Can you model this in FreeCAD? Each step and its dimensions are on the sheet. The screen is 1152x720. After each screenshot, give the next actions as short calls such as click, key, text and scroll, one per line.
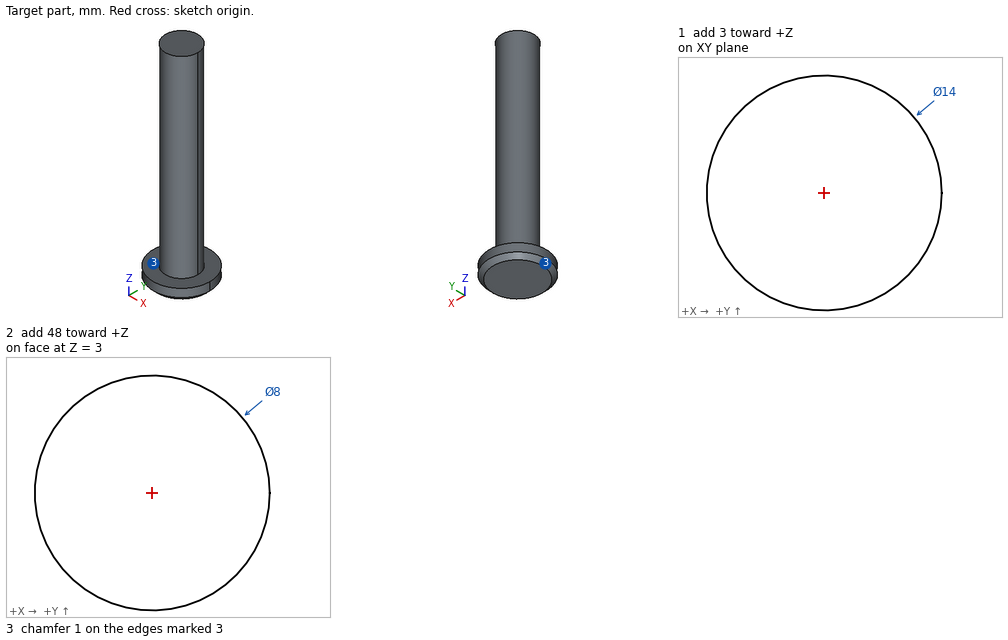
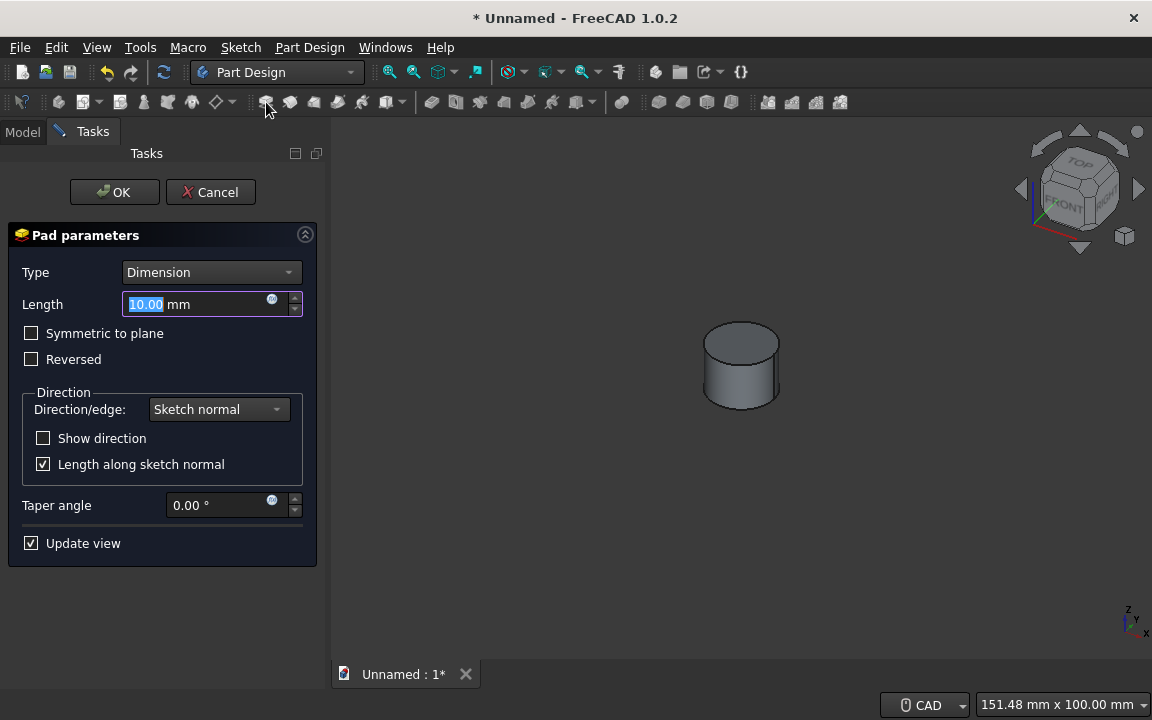
text(3)
key(Tab)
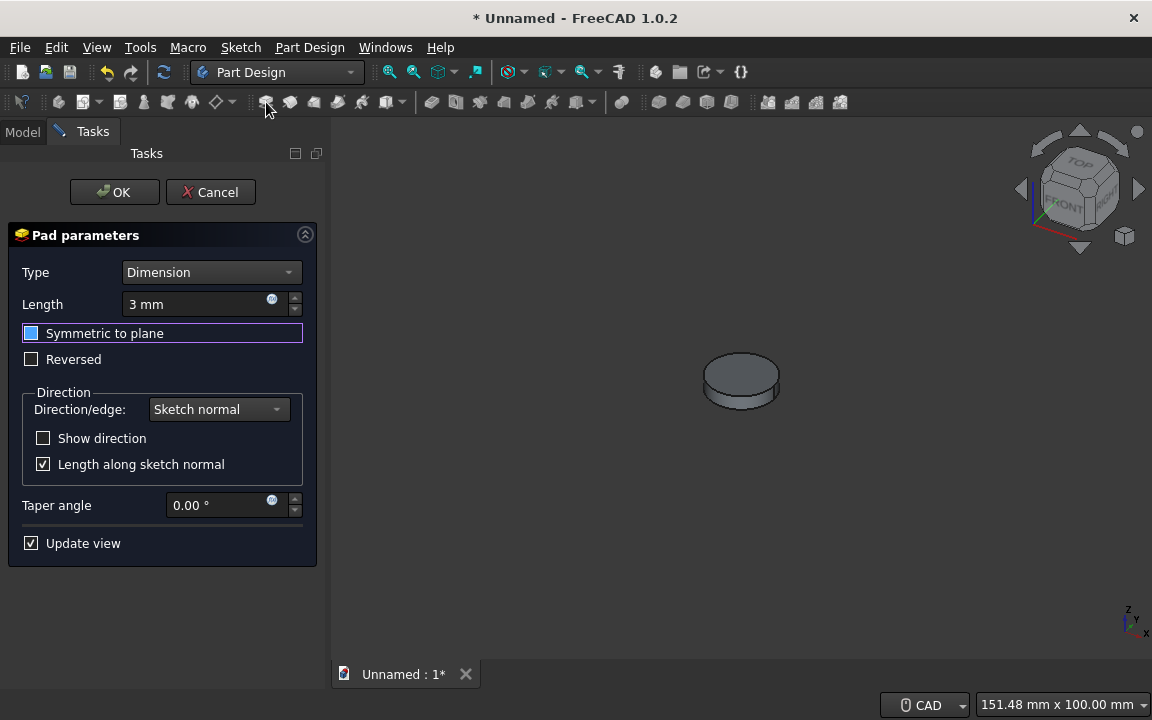
click(115, 192)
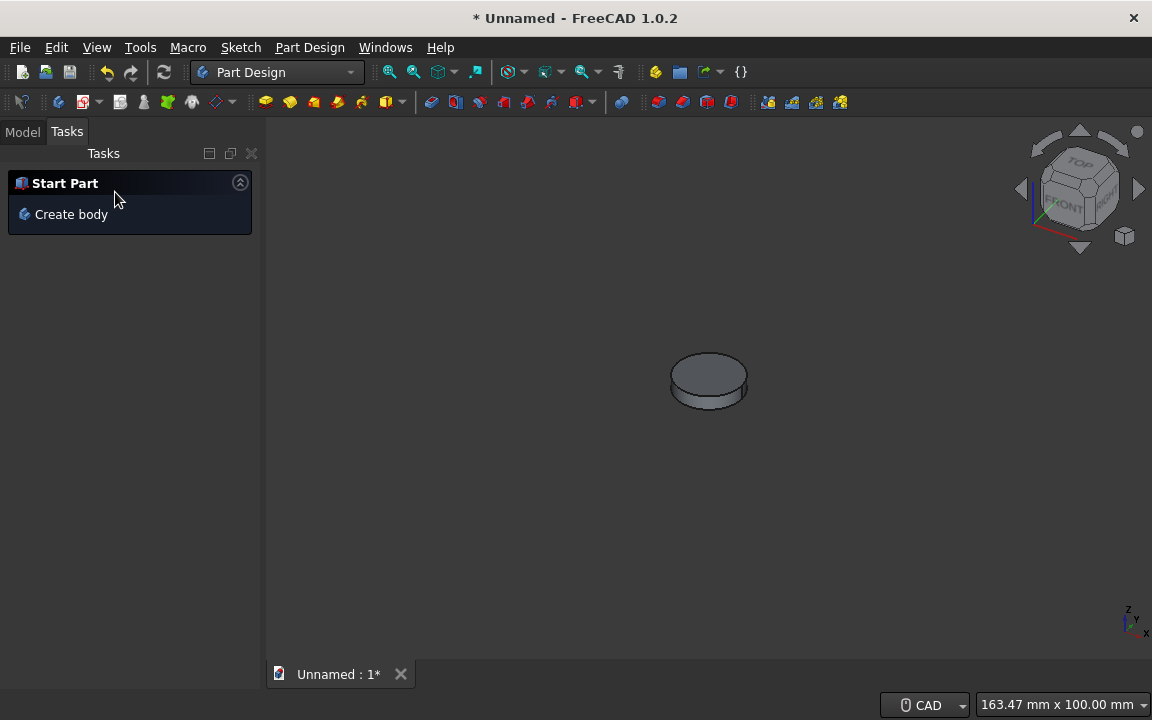
click(390, 72)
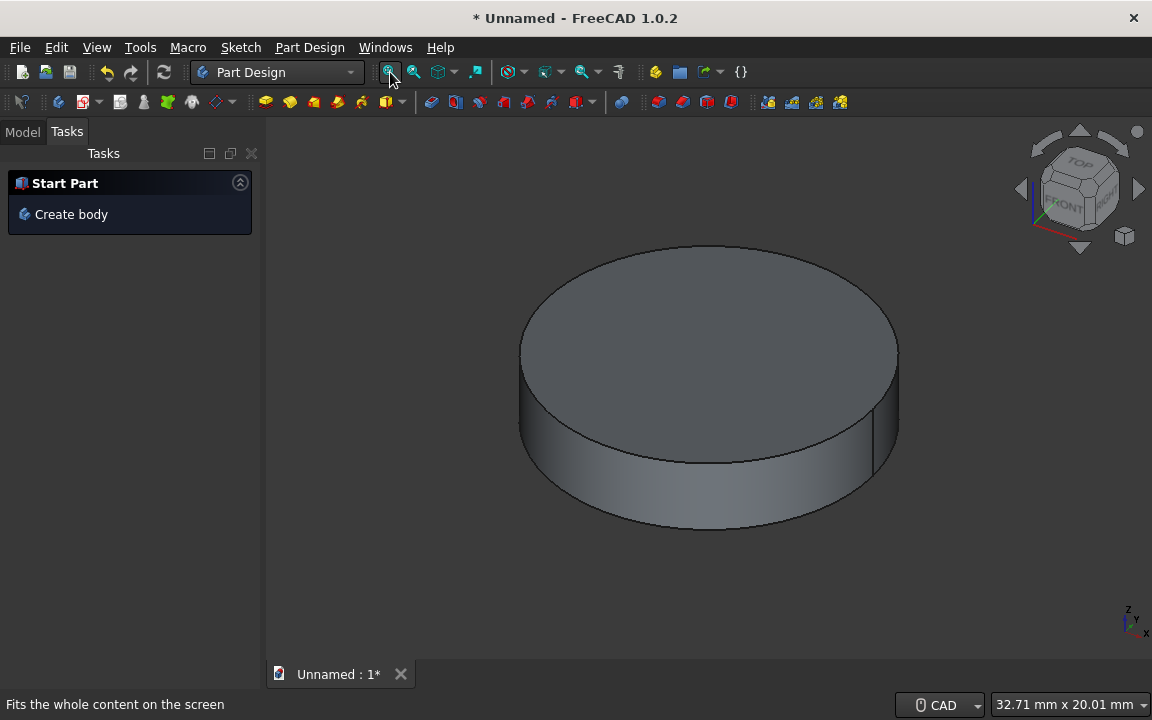
click(709, 354)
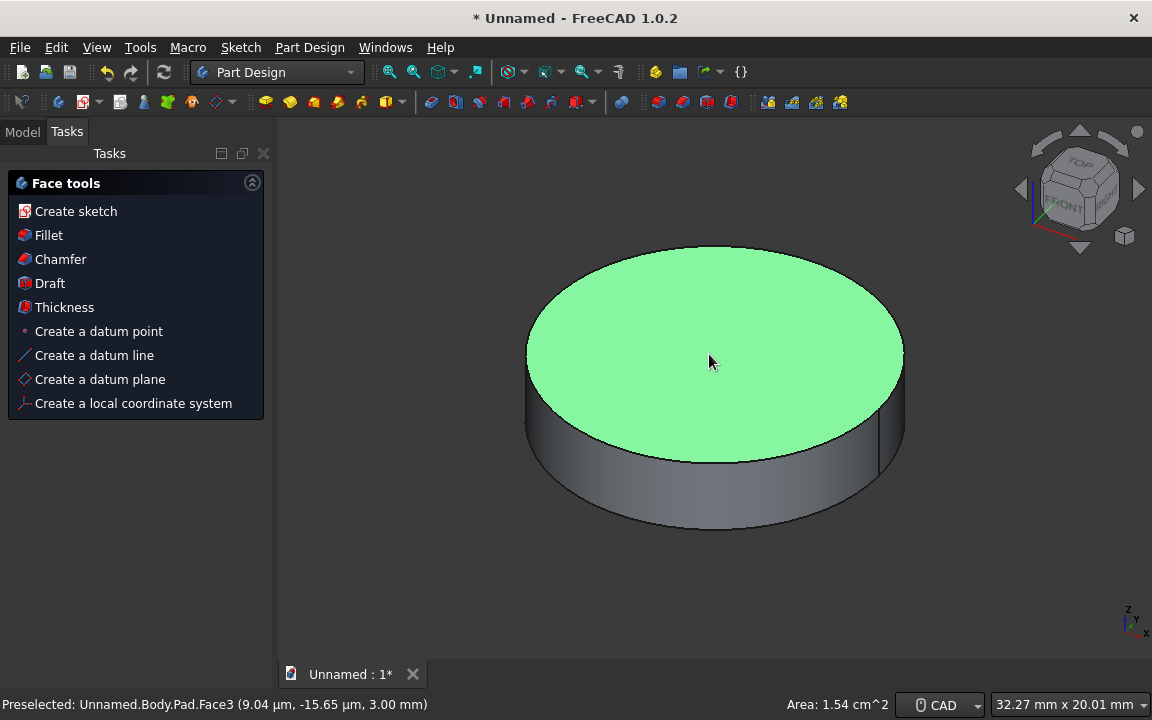
click(84, 102)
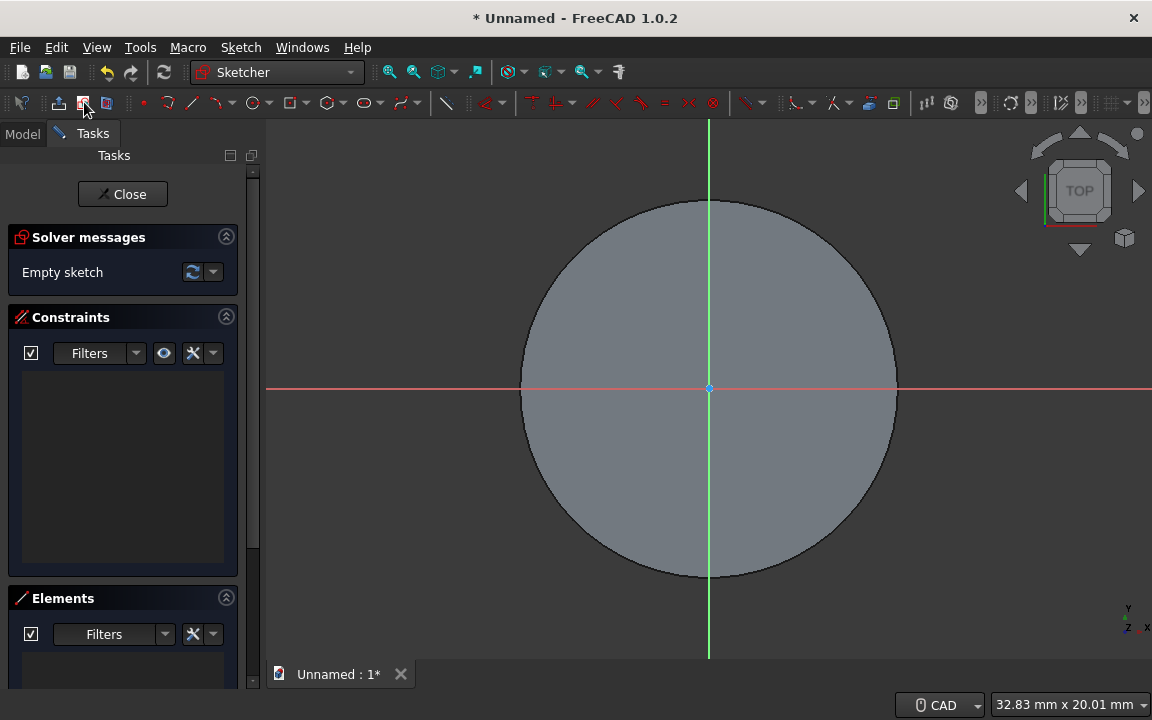
scroll(848, 389, up, 2)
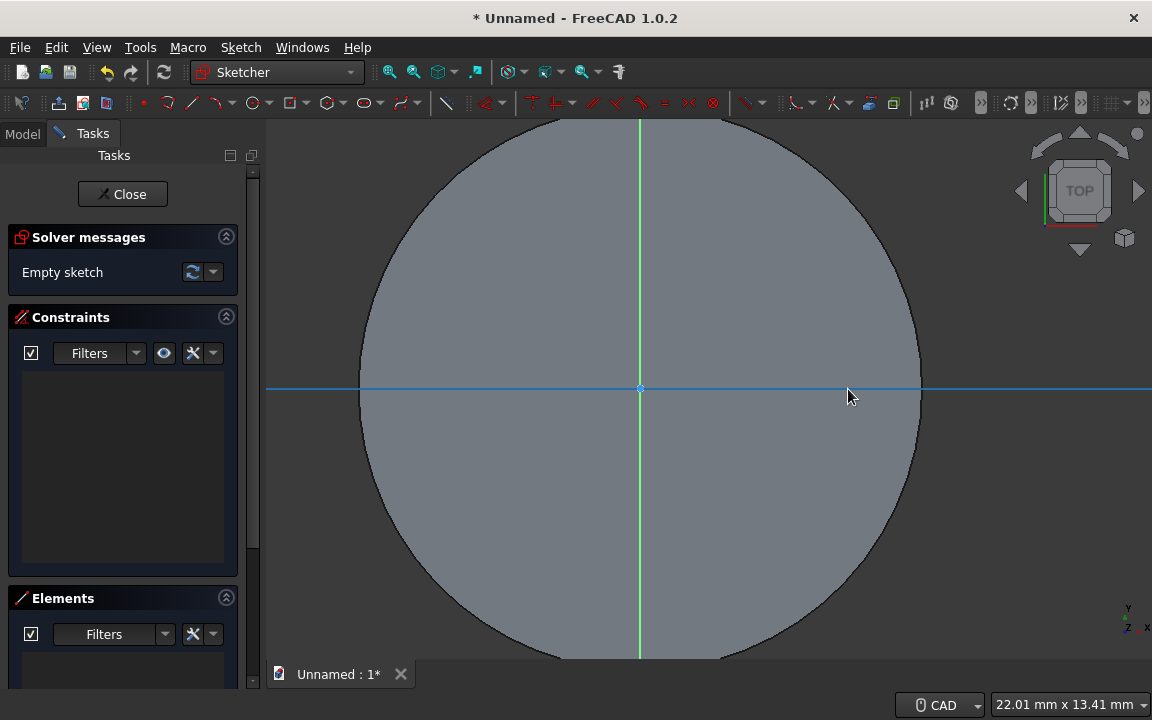
click(254, 104)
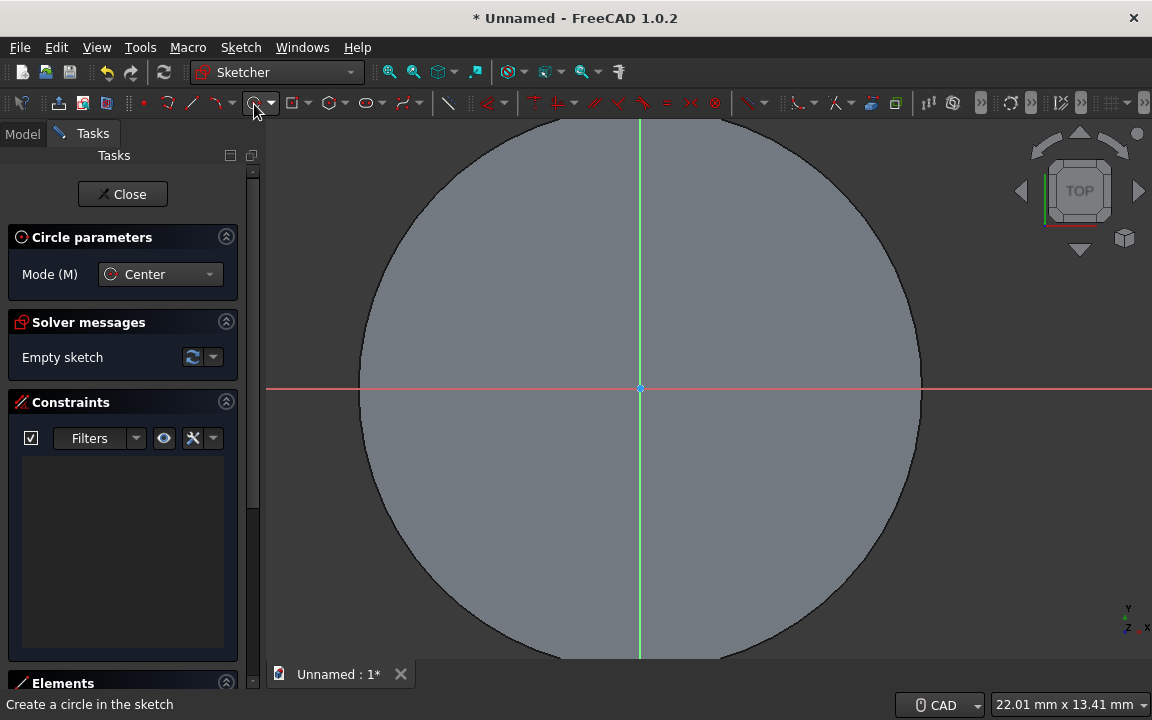
click(640, 389)
click(754, 275)
key(Escape)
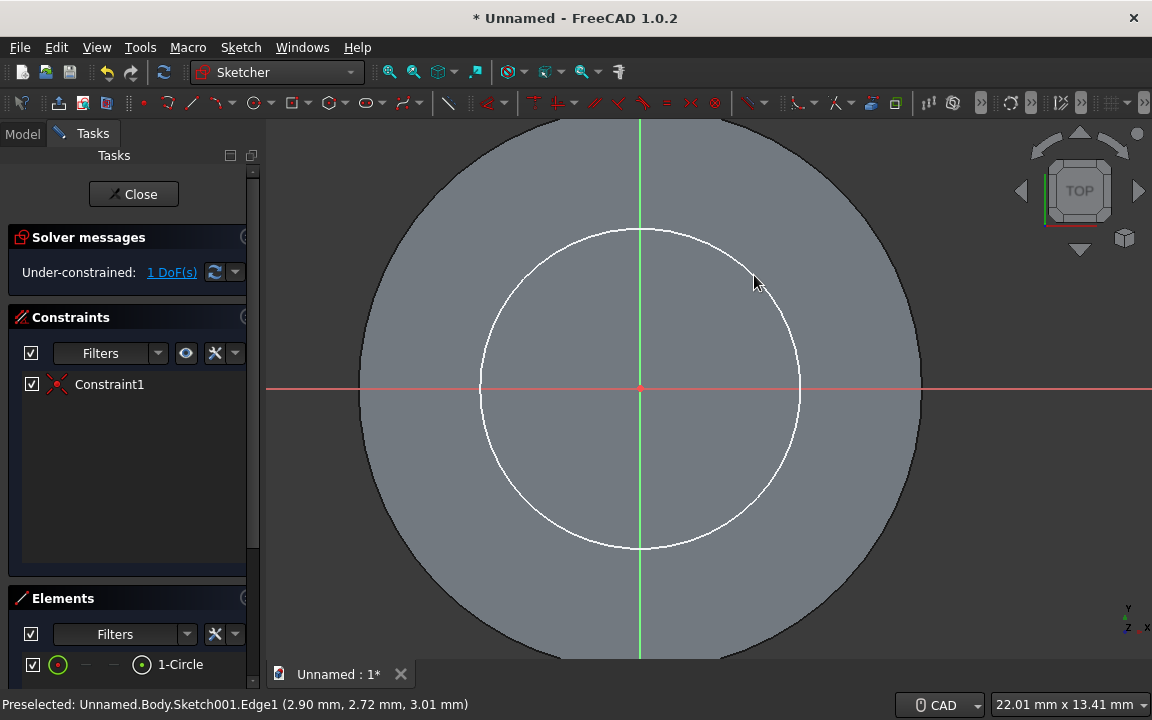
click(753, 275)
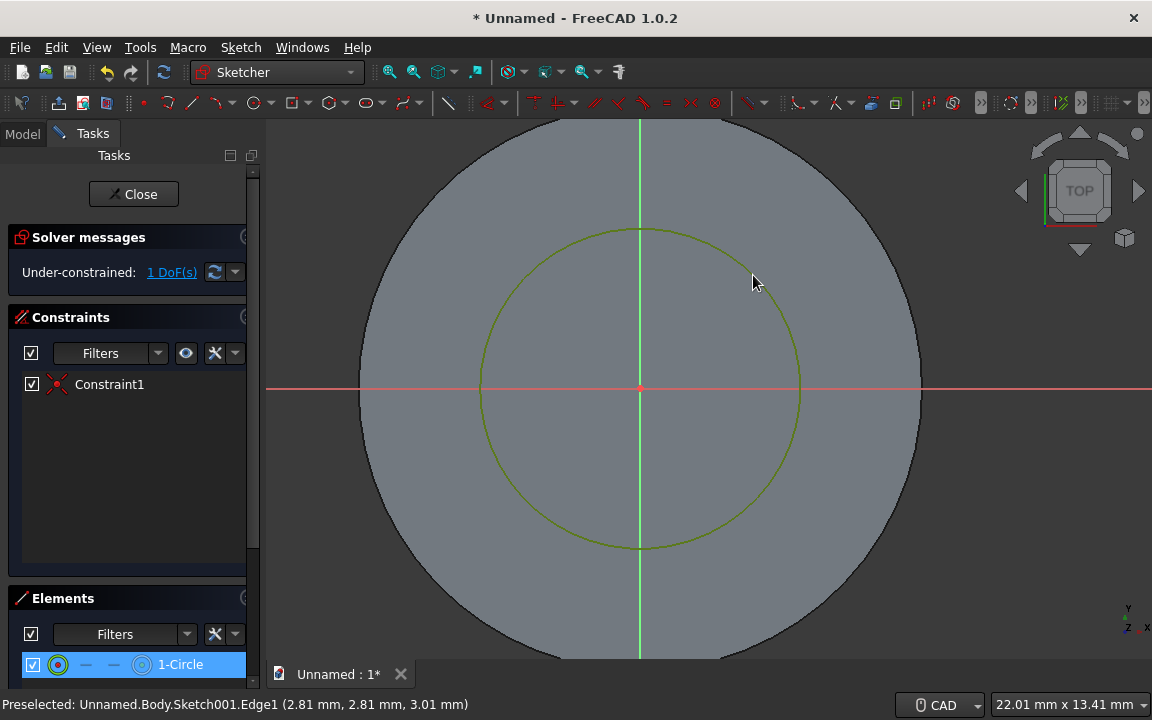
click(506, 104)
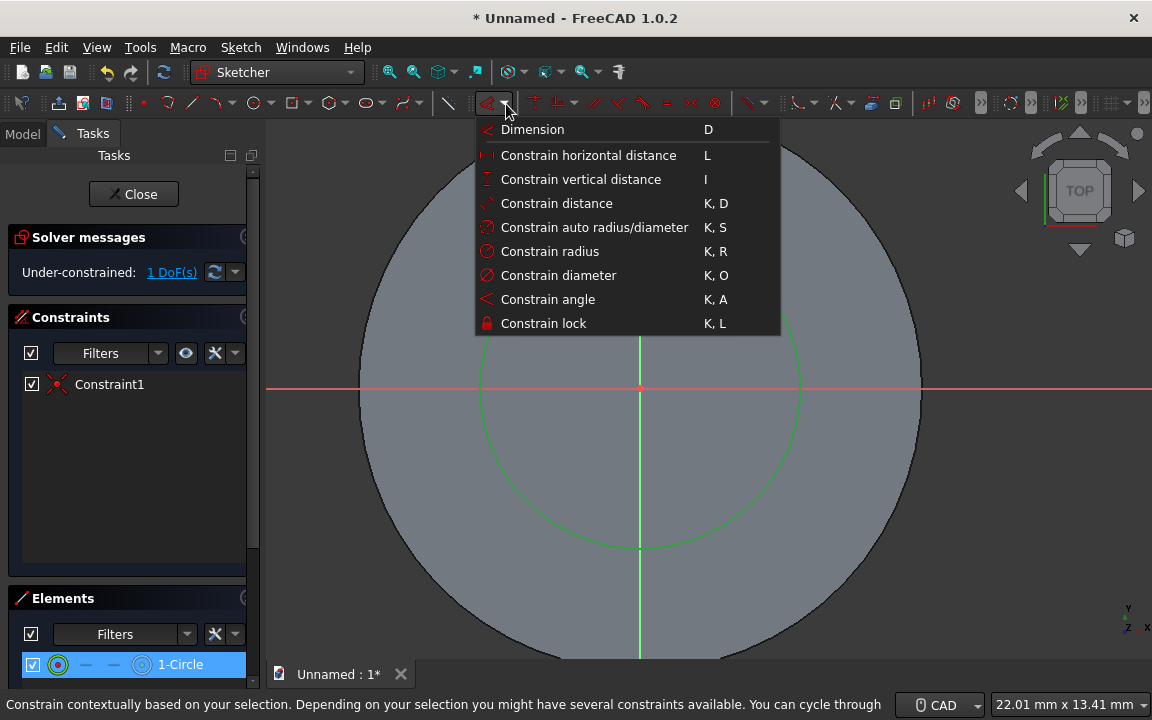
click(628, 275)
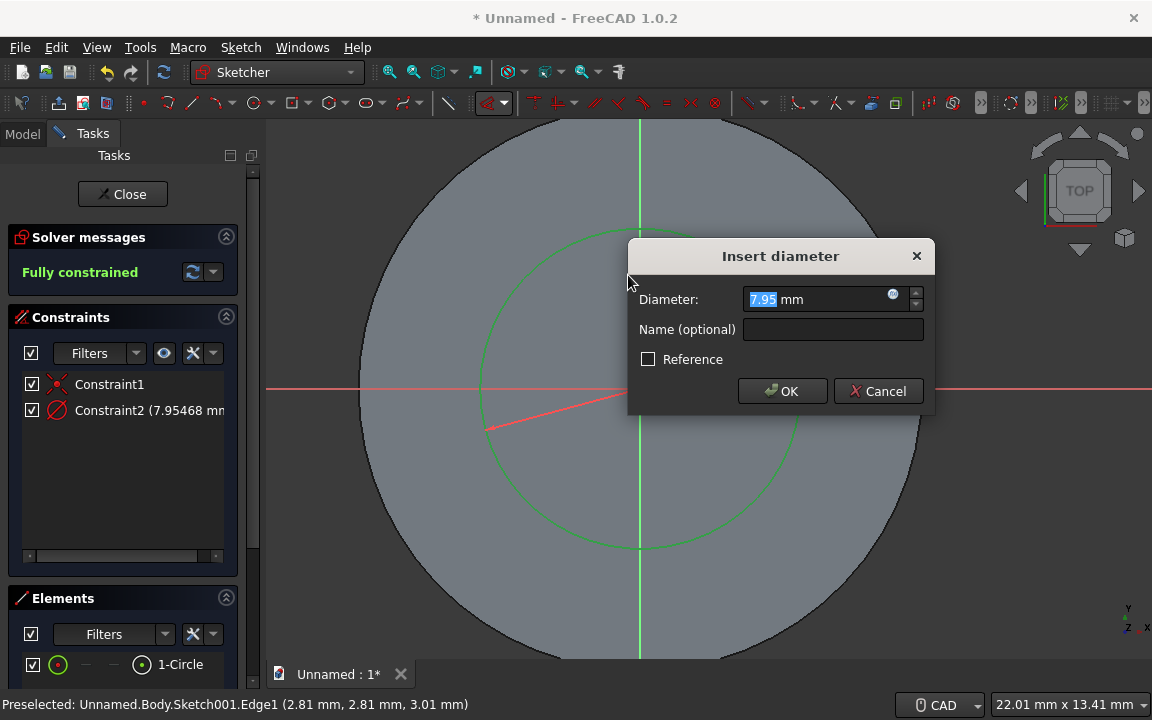
text(8)
key(Return)